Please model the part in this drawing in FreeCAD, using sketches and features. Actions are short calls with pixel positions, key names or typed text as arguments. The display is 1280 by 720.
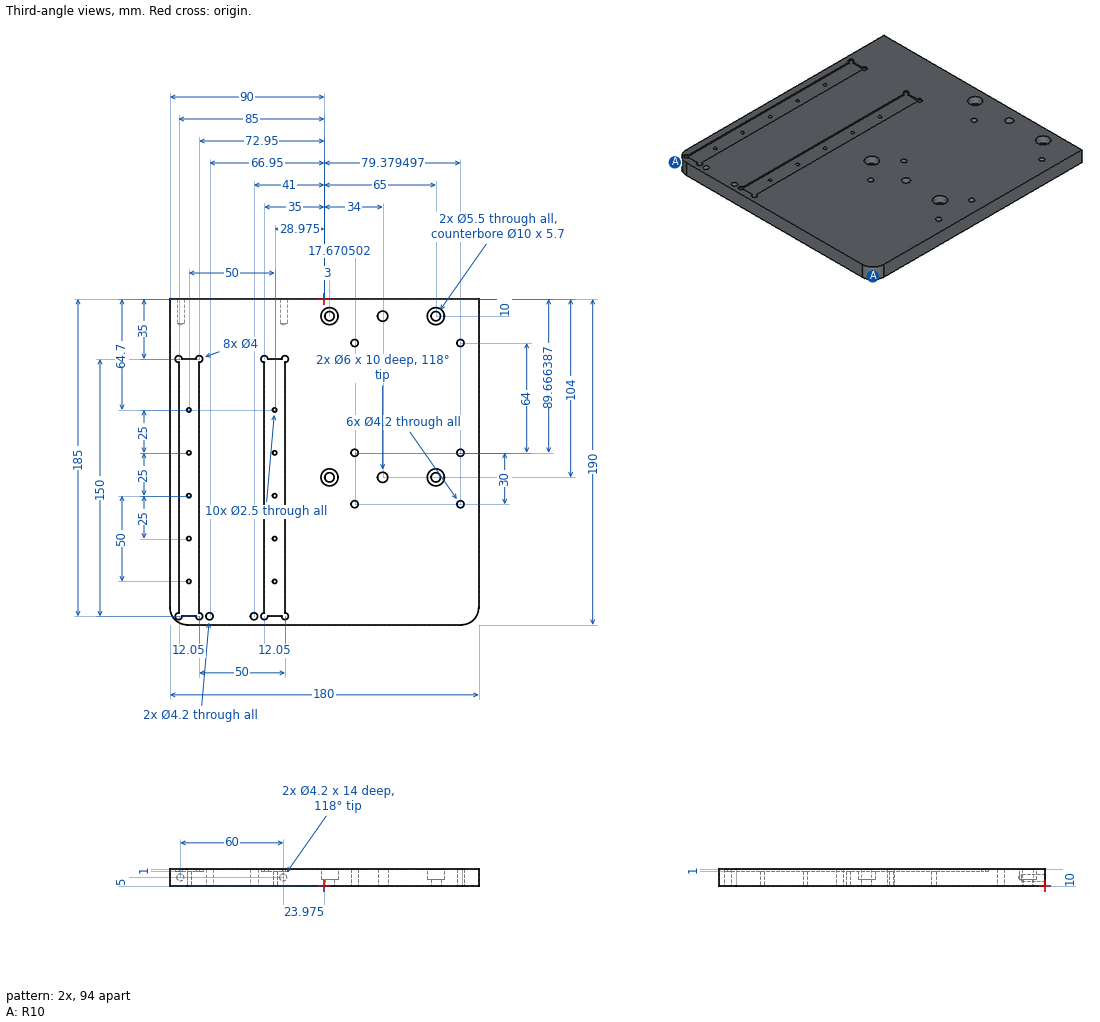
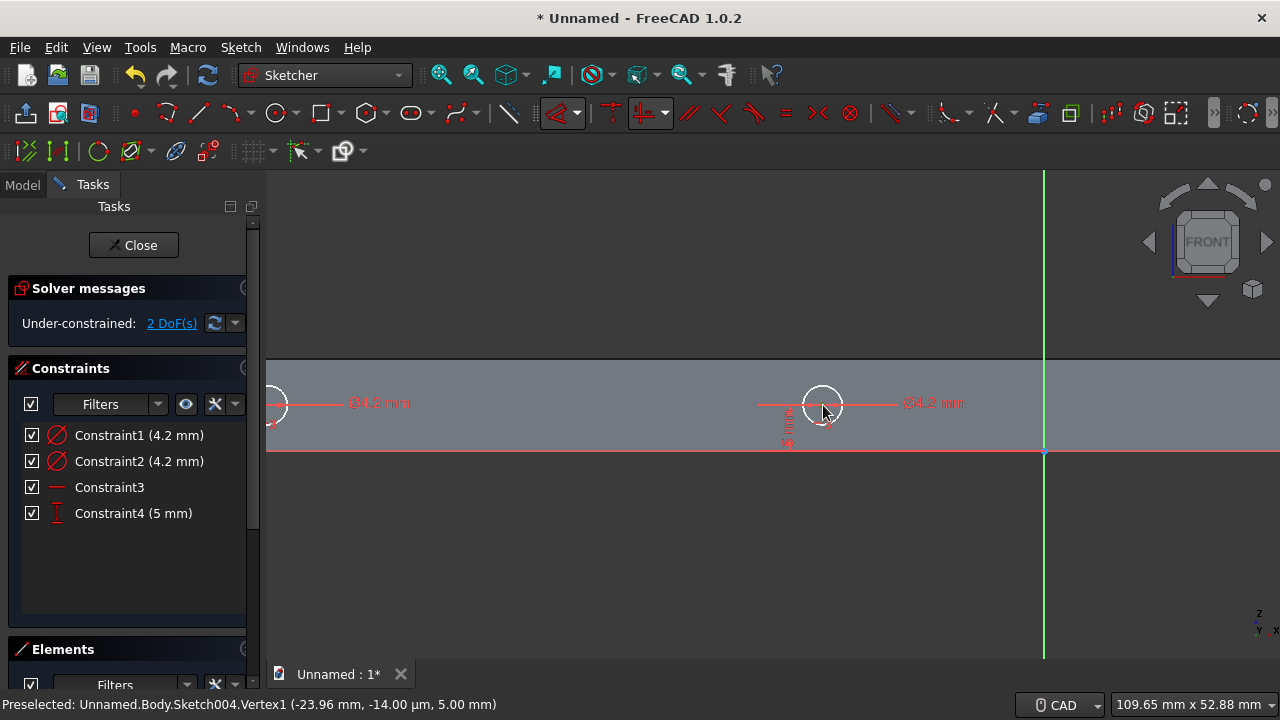
scroll(823, 406, down, 2)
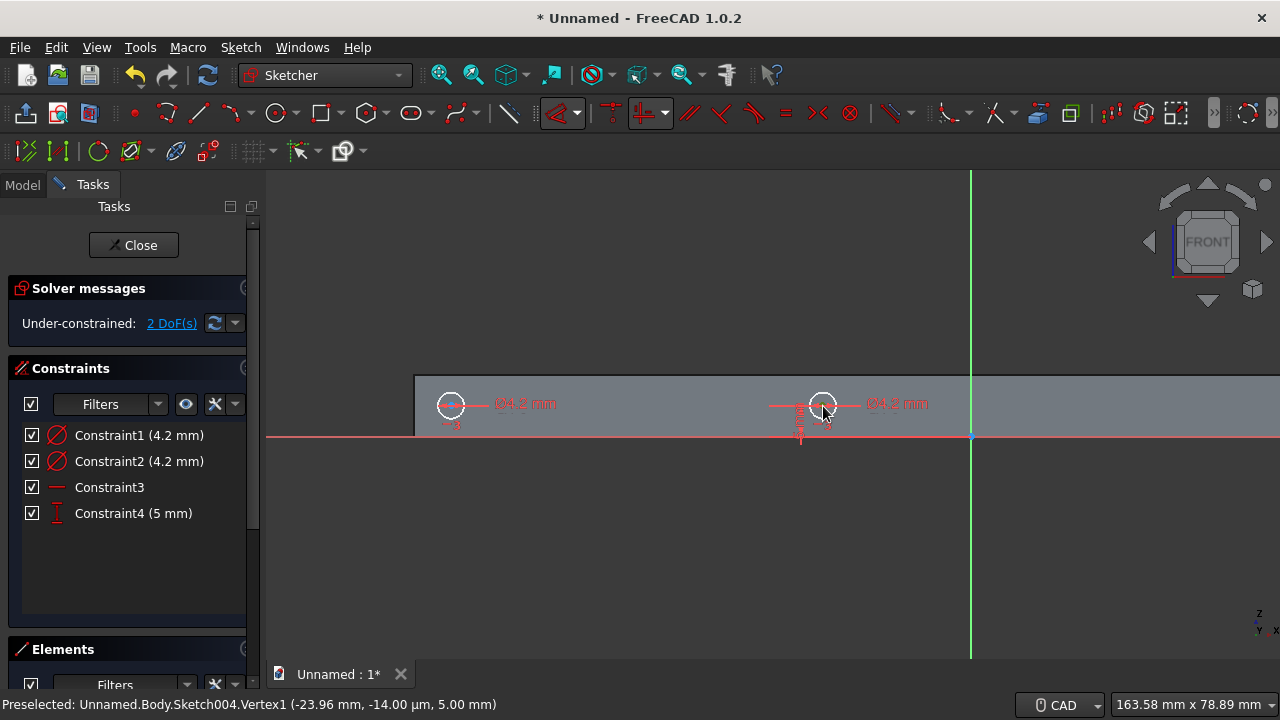
click(451, 406)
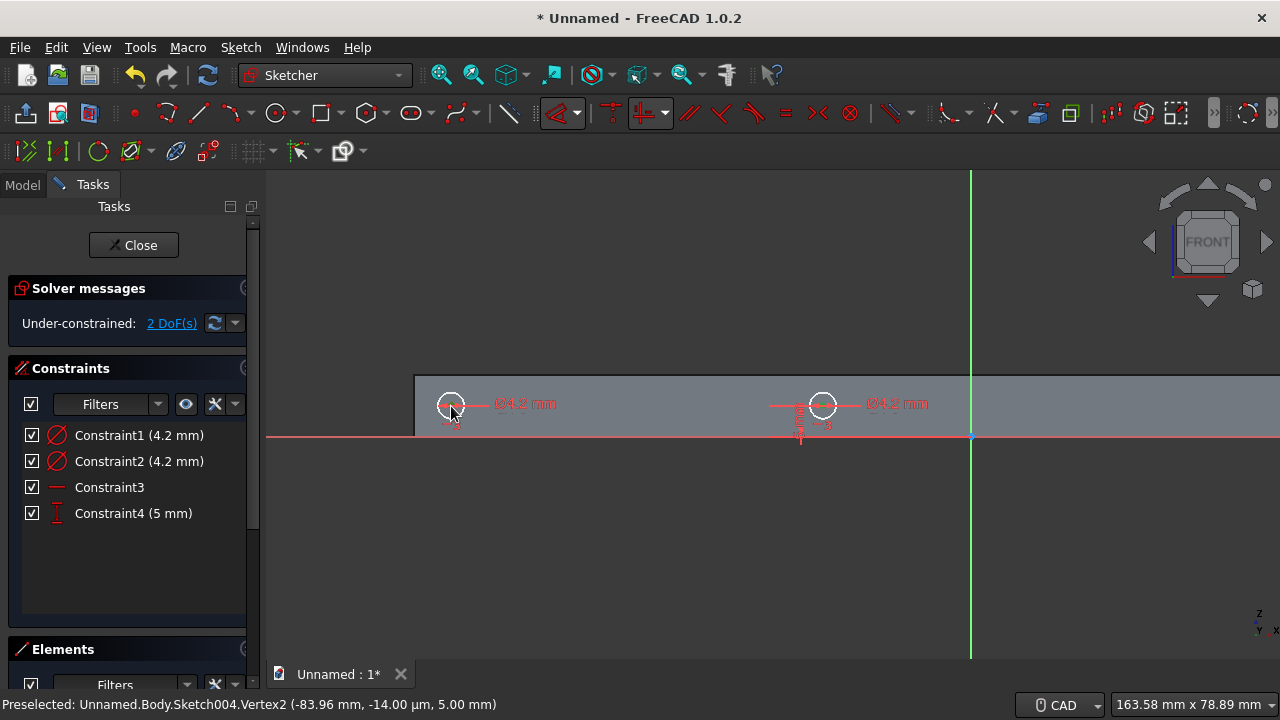
key(l)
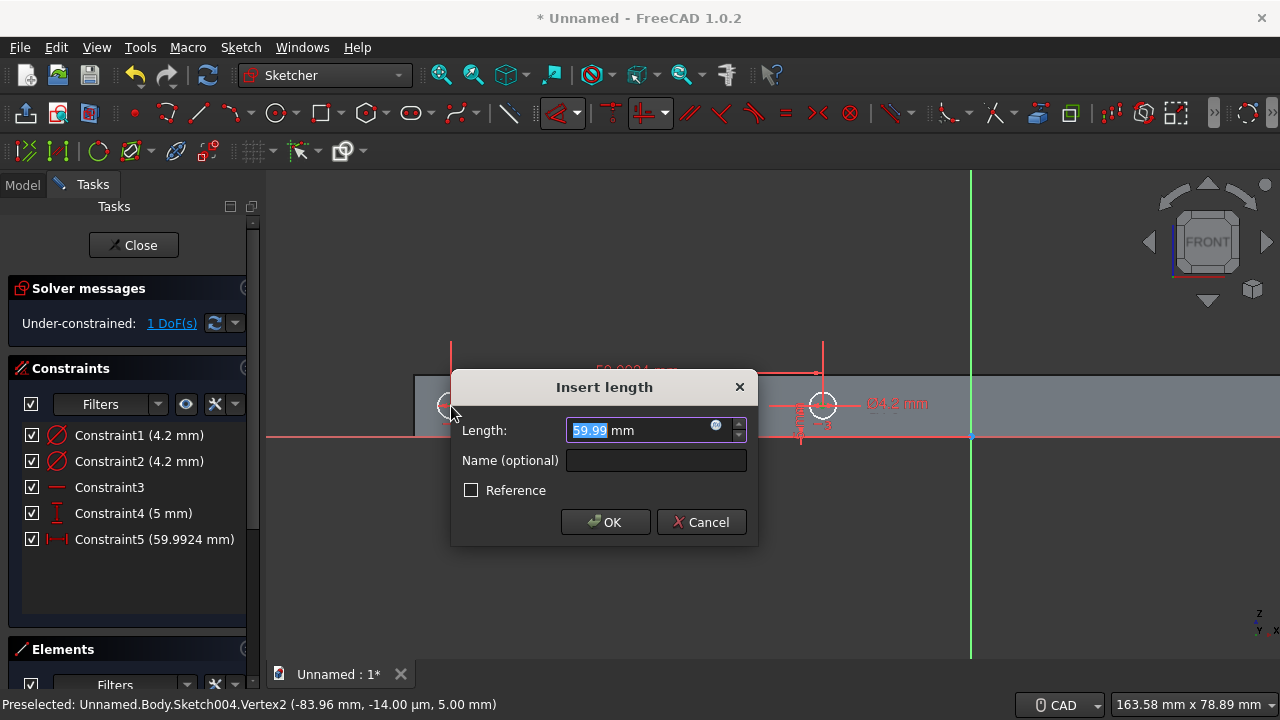
text(60)
key(Return)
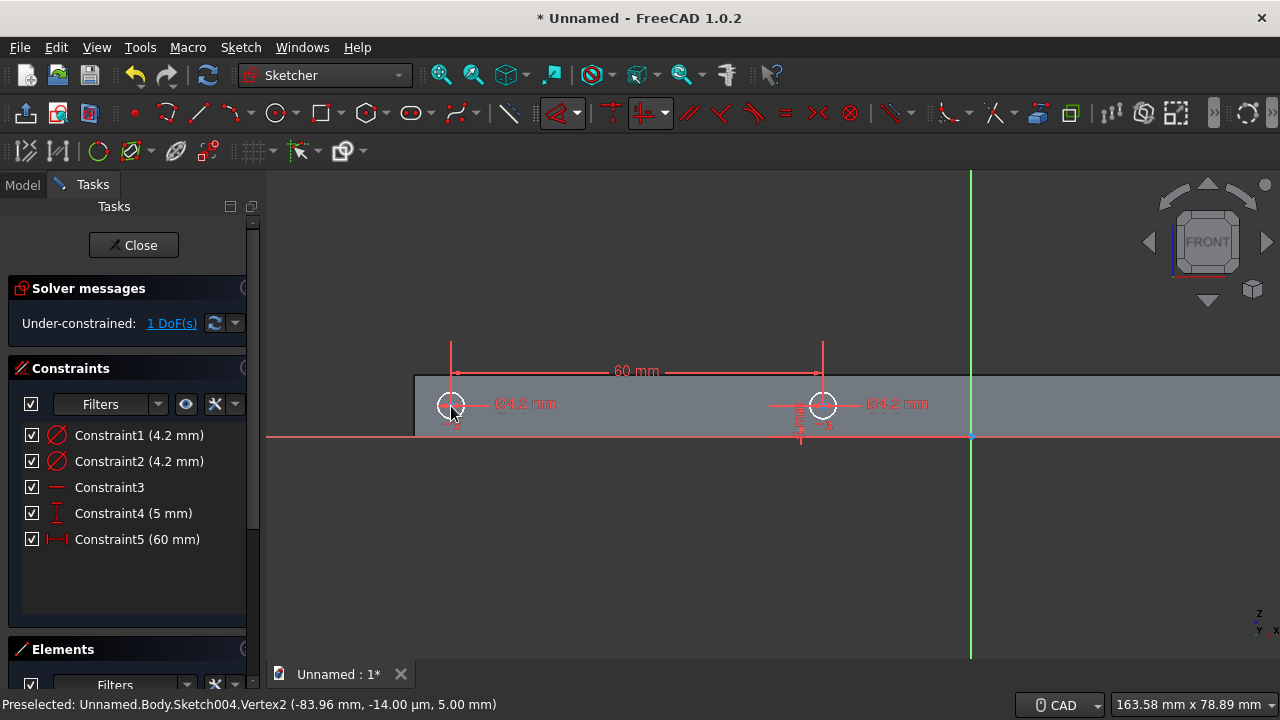
click(823, 406)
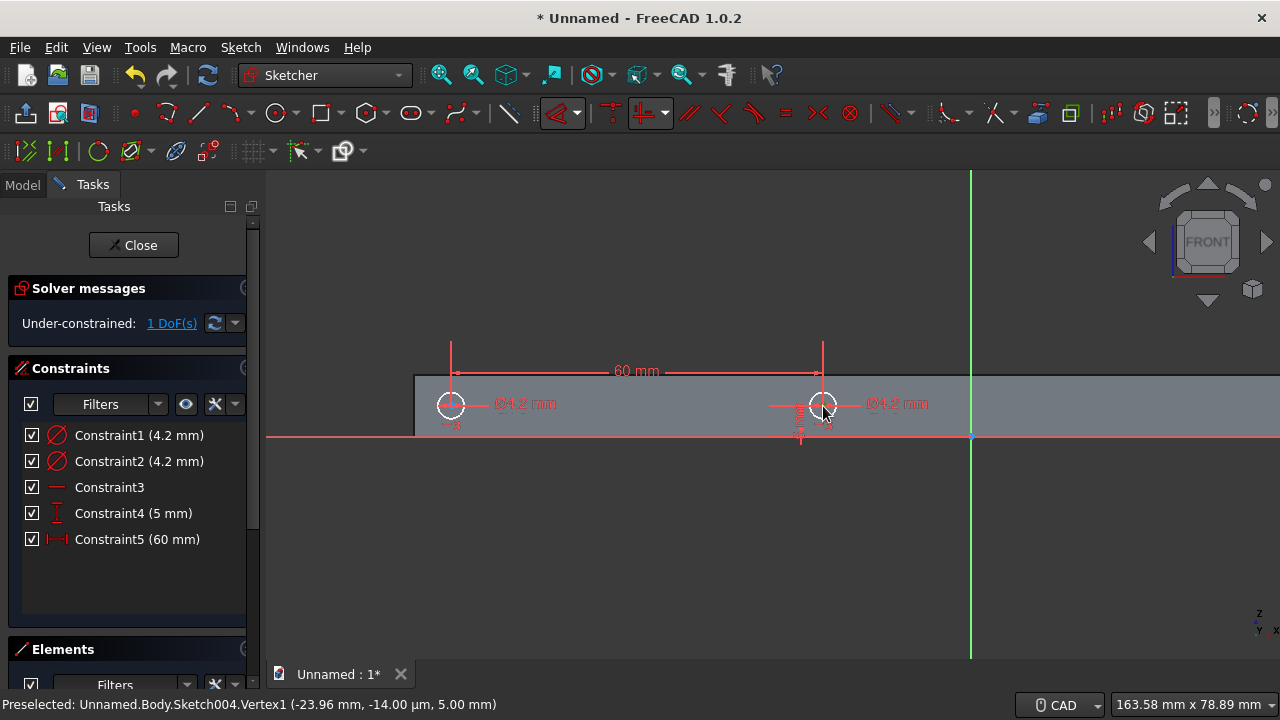
key(l)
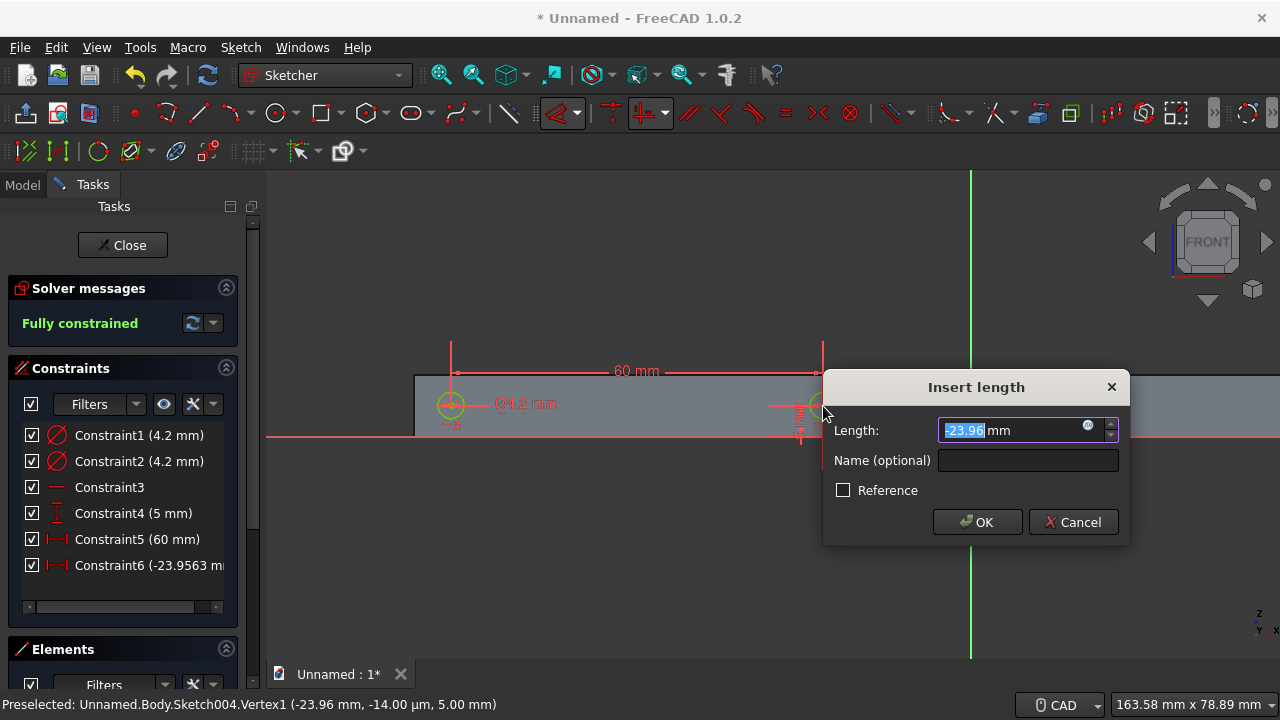
text(-23.975)
key(Return)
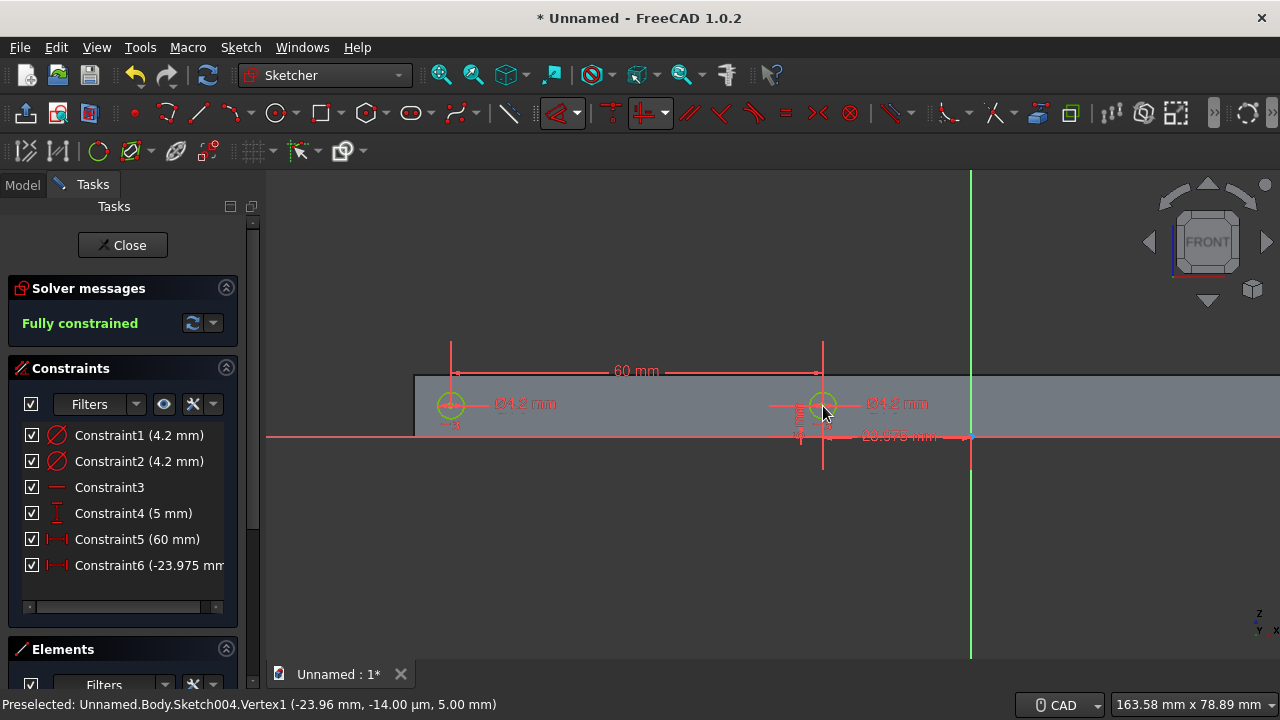
click(123, 245)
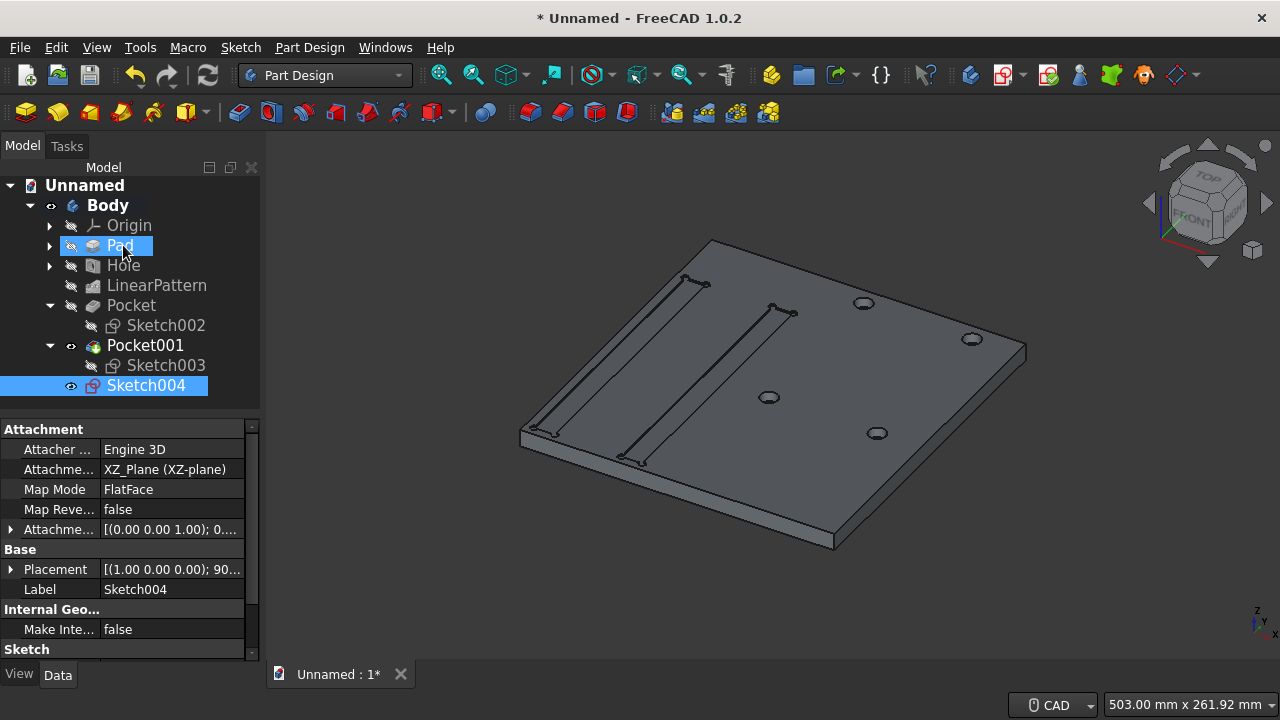
click(272, 112)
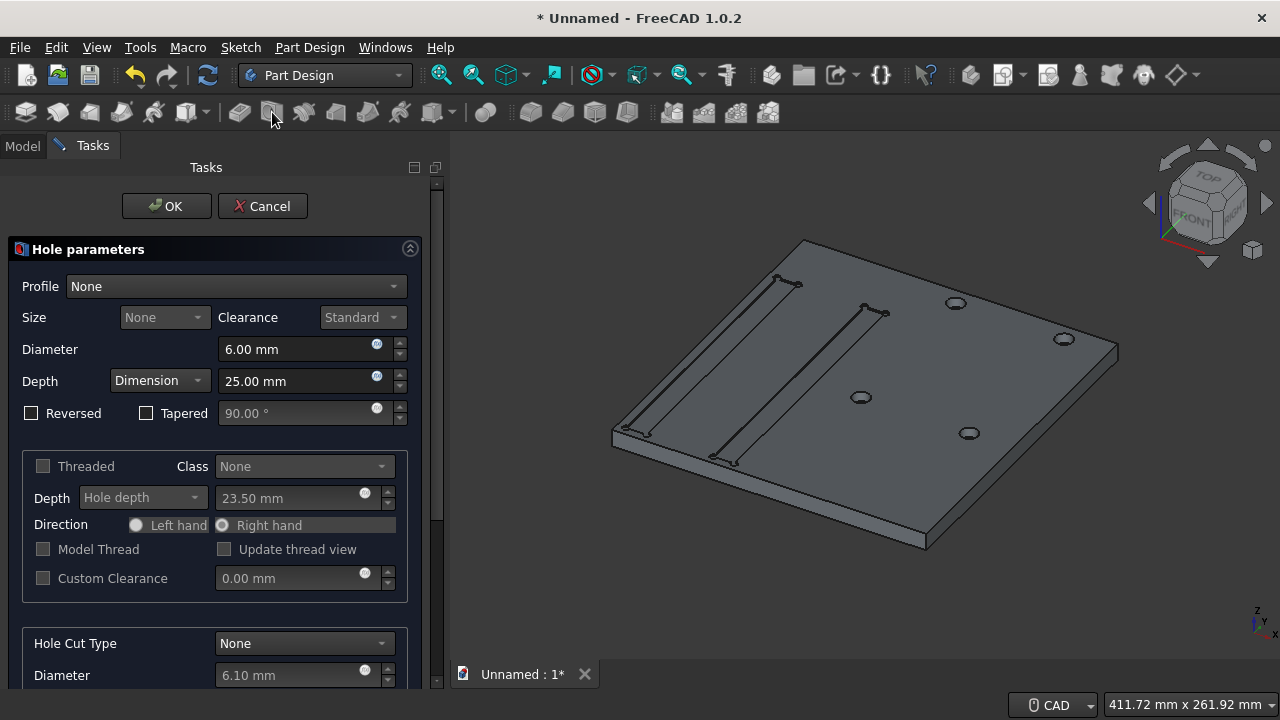
triple_click(305, 349)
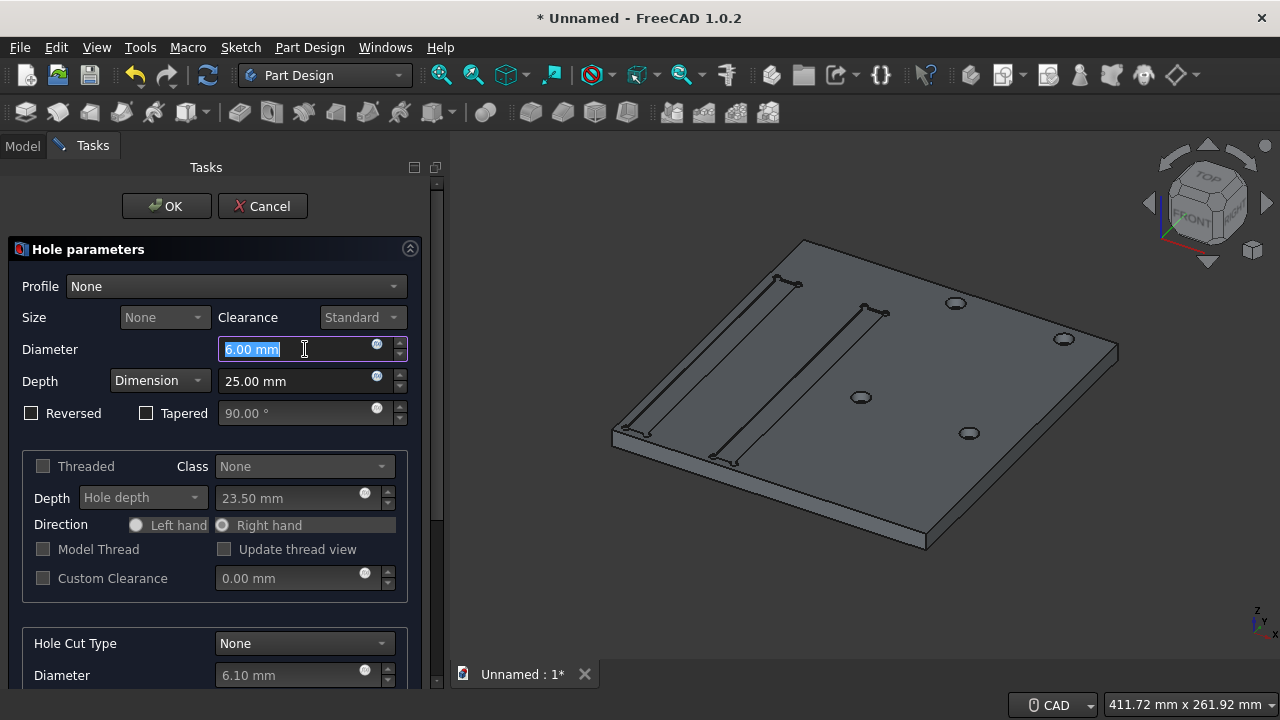
text(4.2)
key(Tab)